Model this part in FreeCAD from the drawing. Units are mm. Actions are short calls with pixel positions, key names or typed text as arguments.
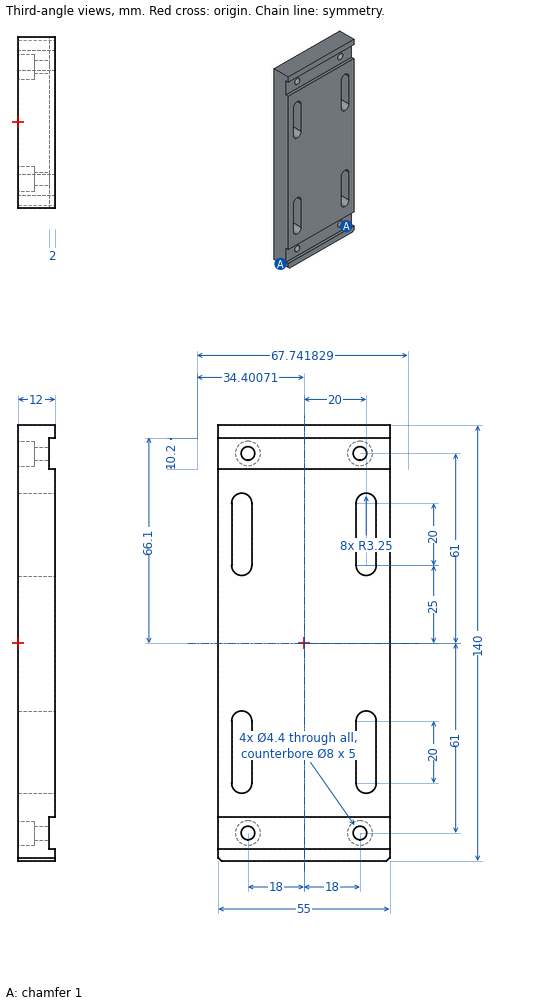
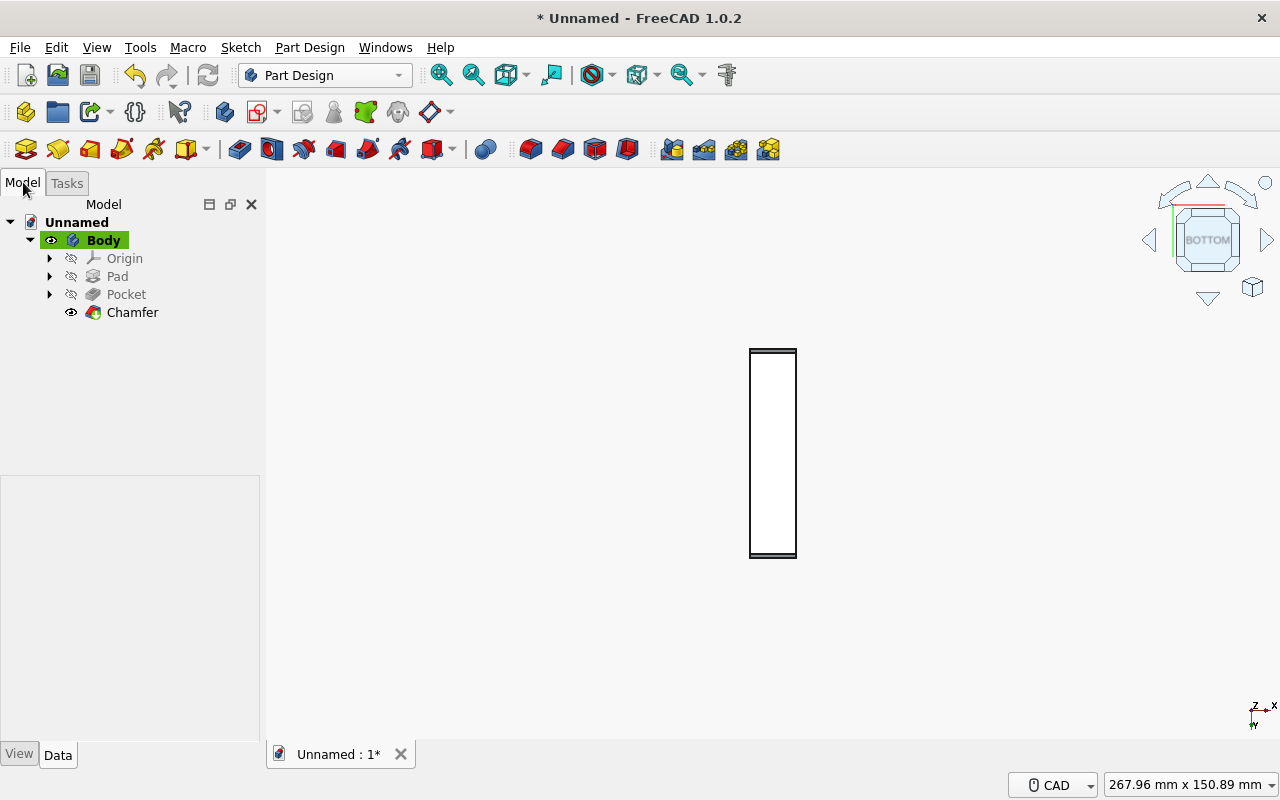
click(116, 294)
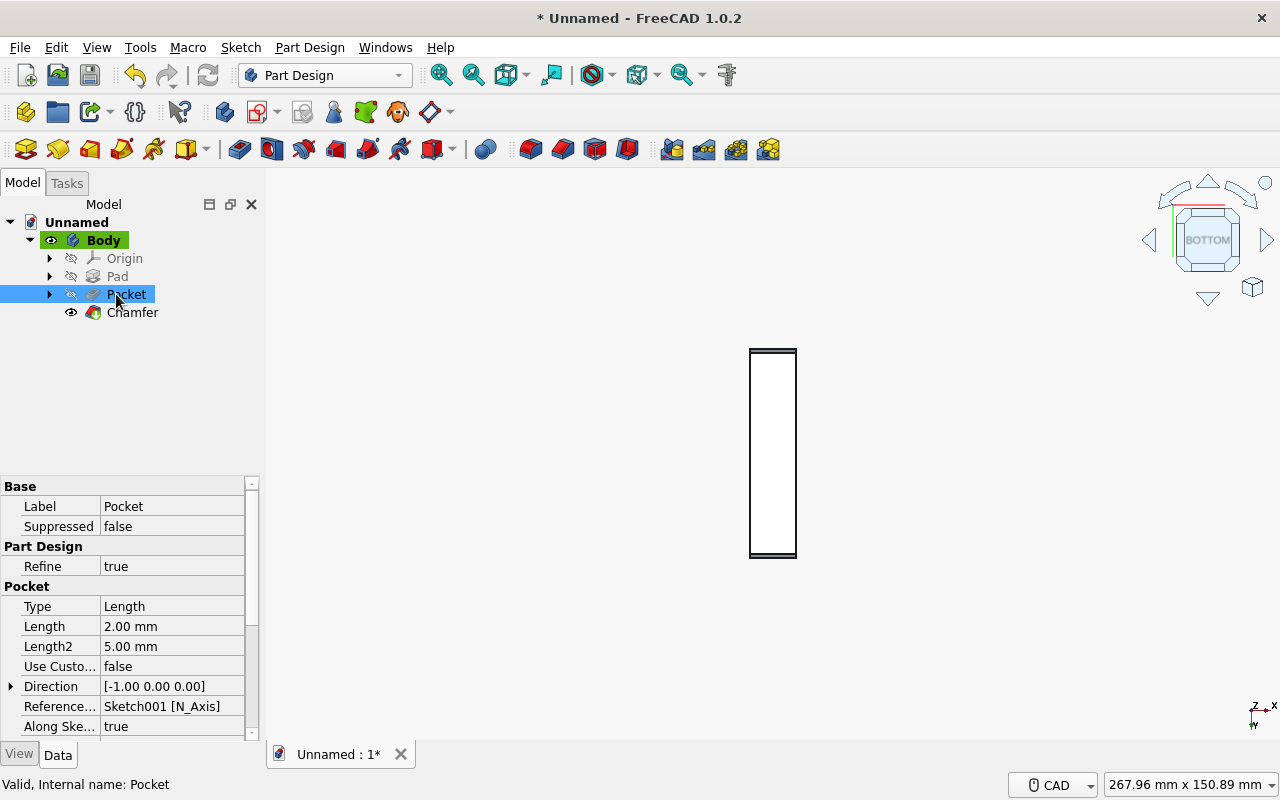
click(672, 150)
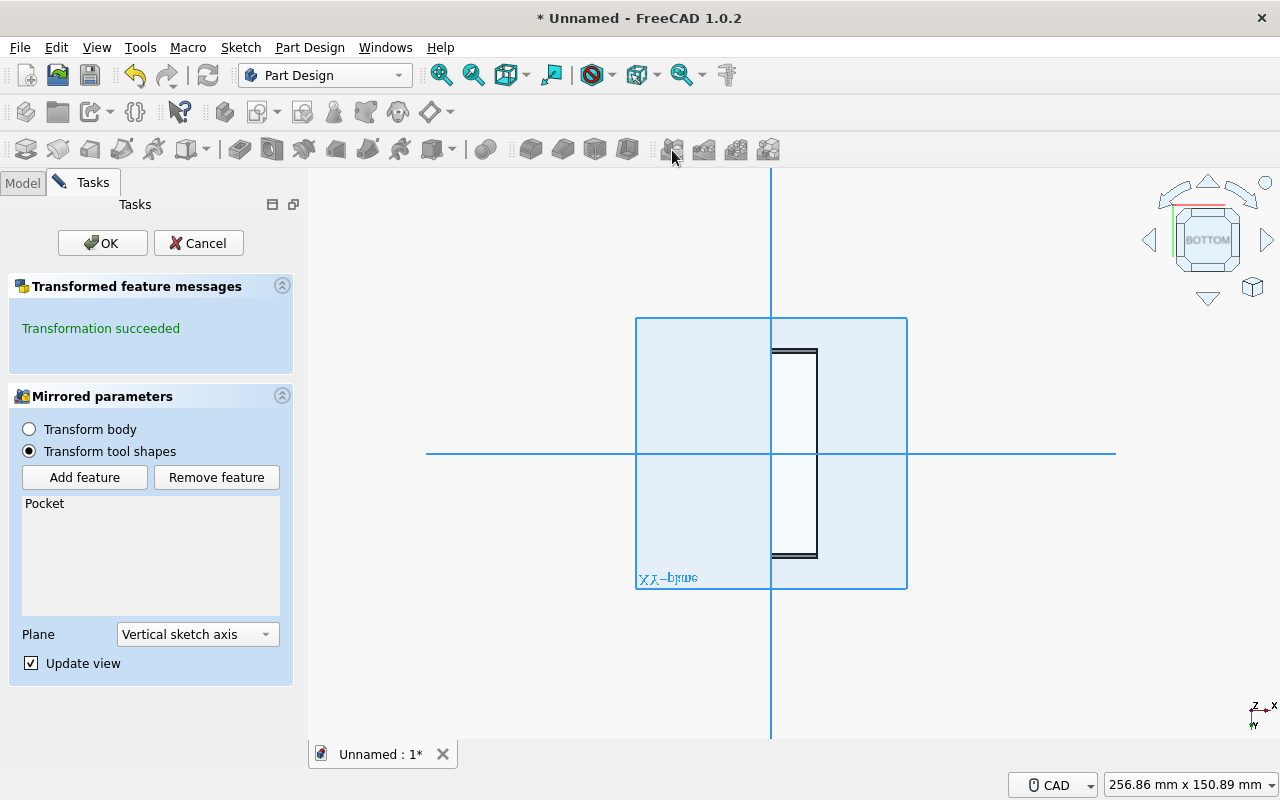
click(198, 634)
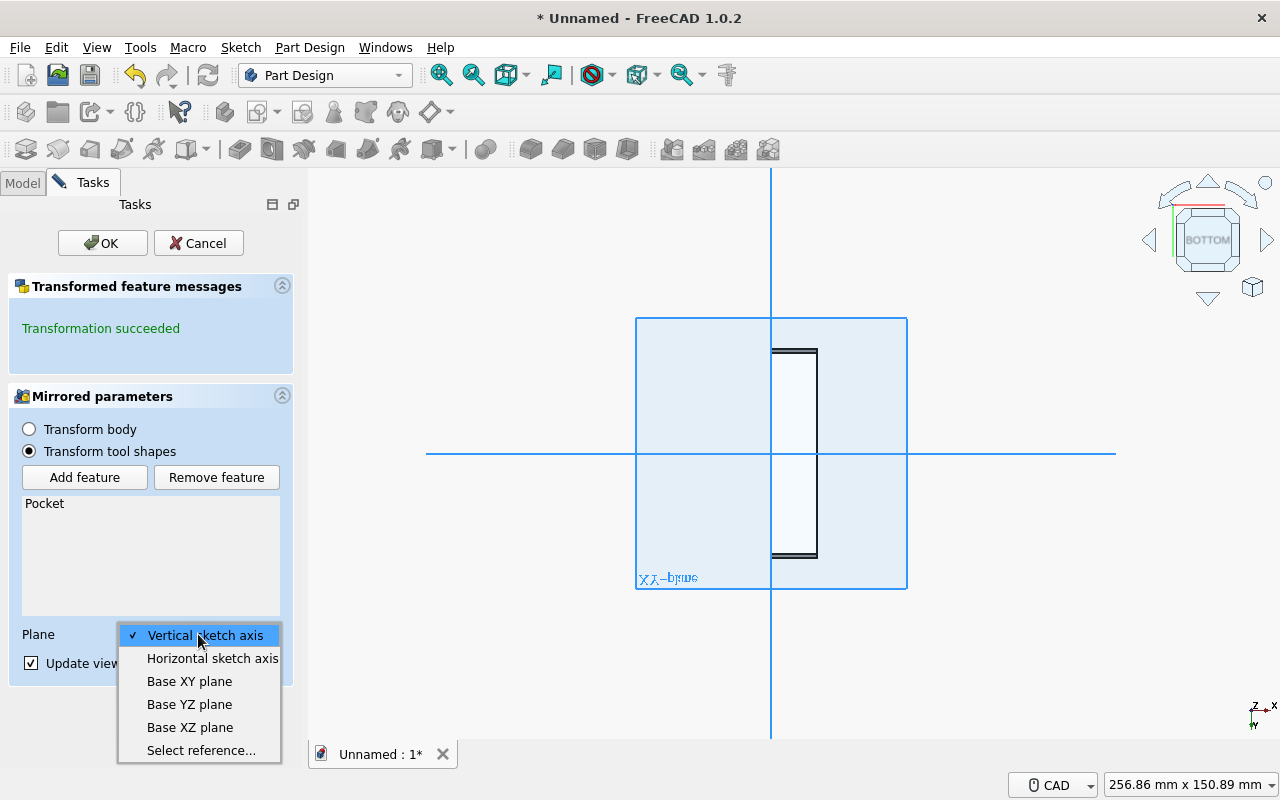
click(198, 682)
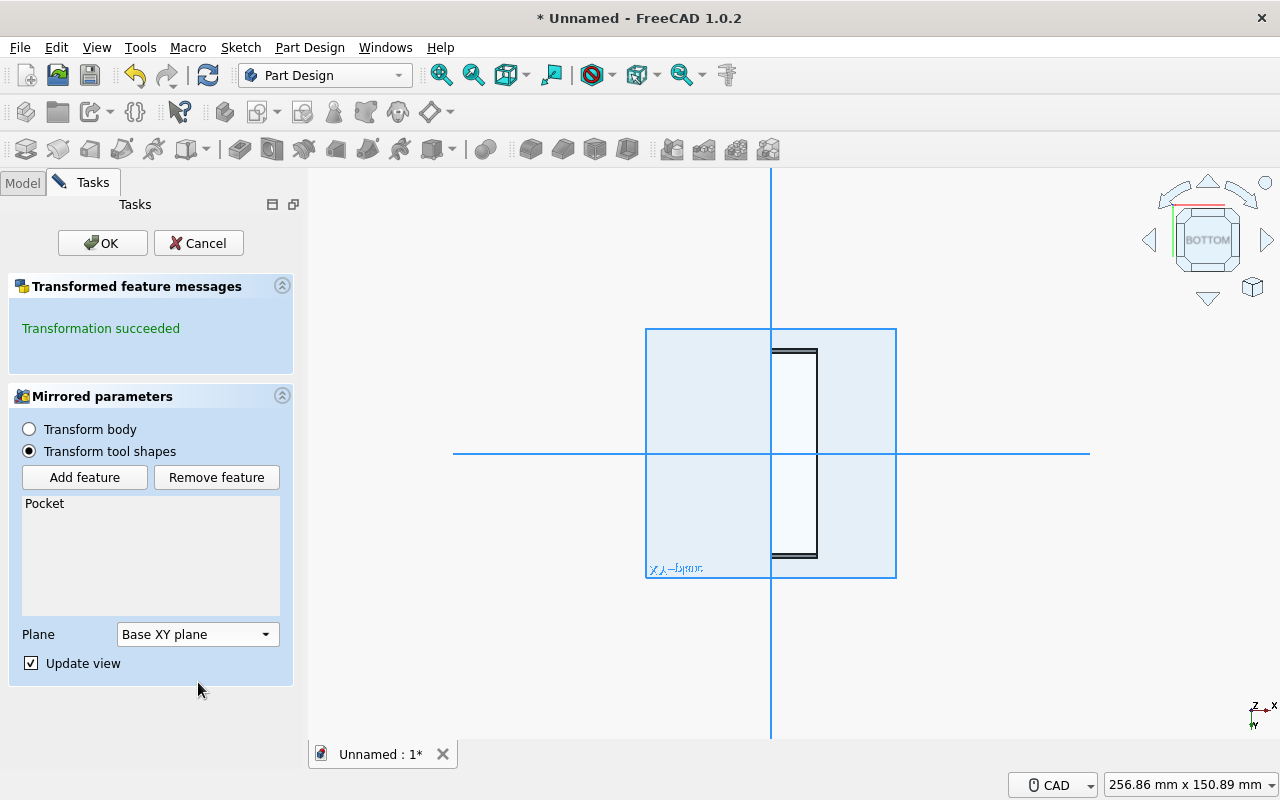
click(103, 243)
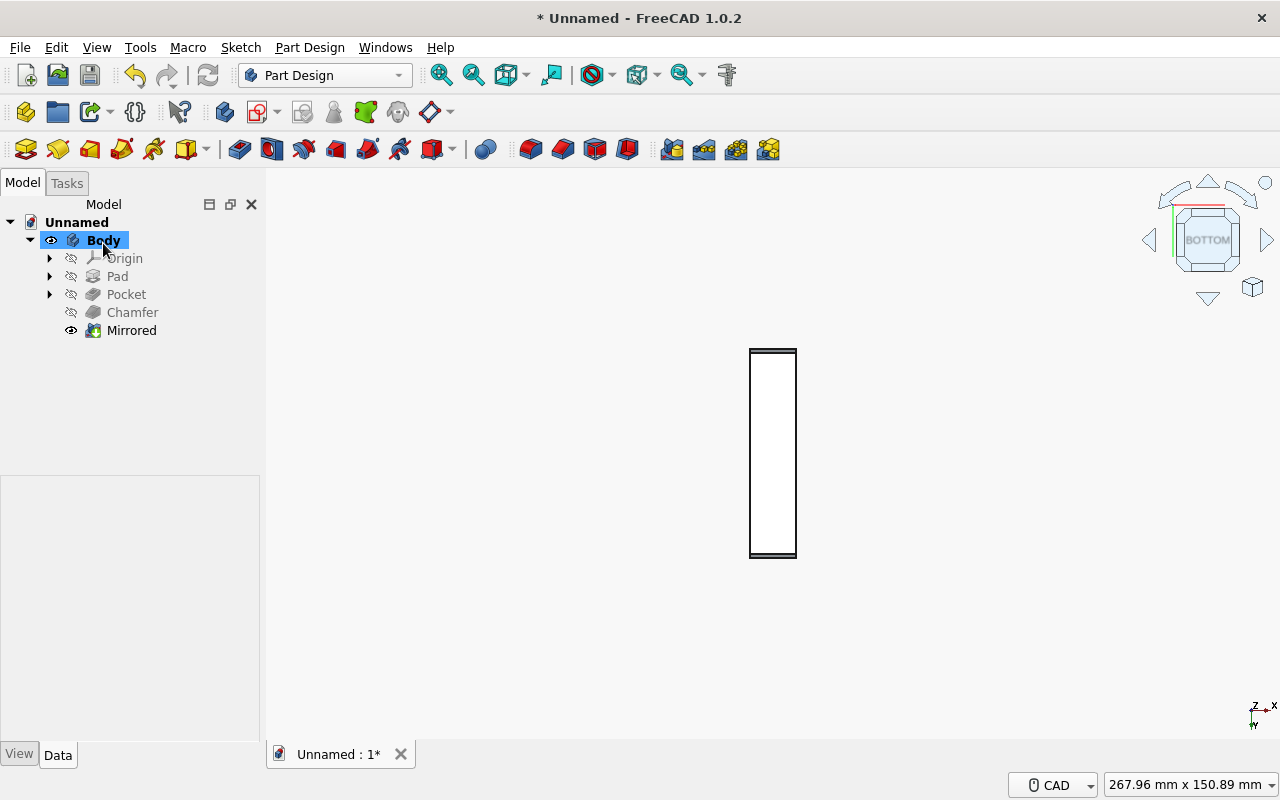
click(442, 76)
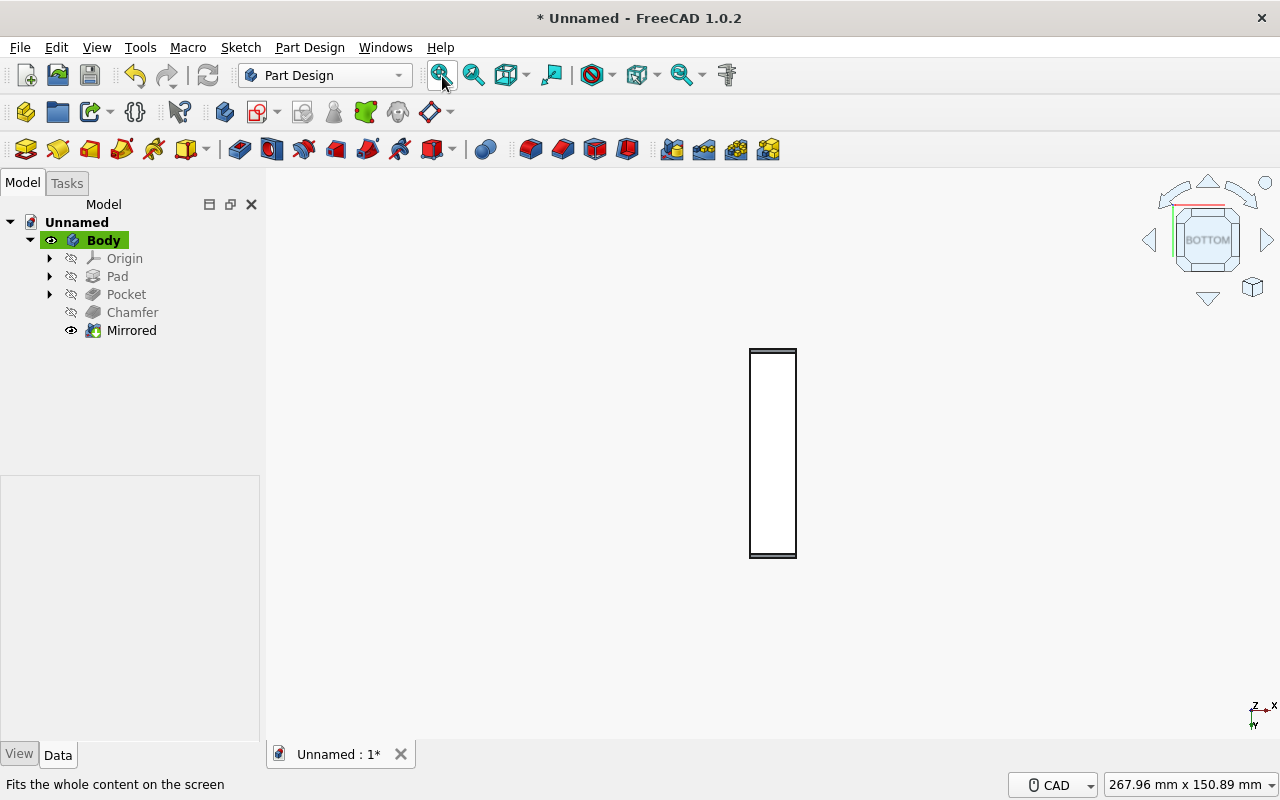
key(0)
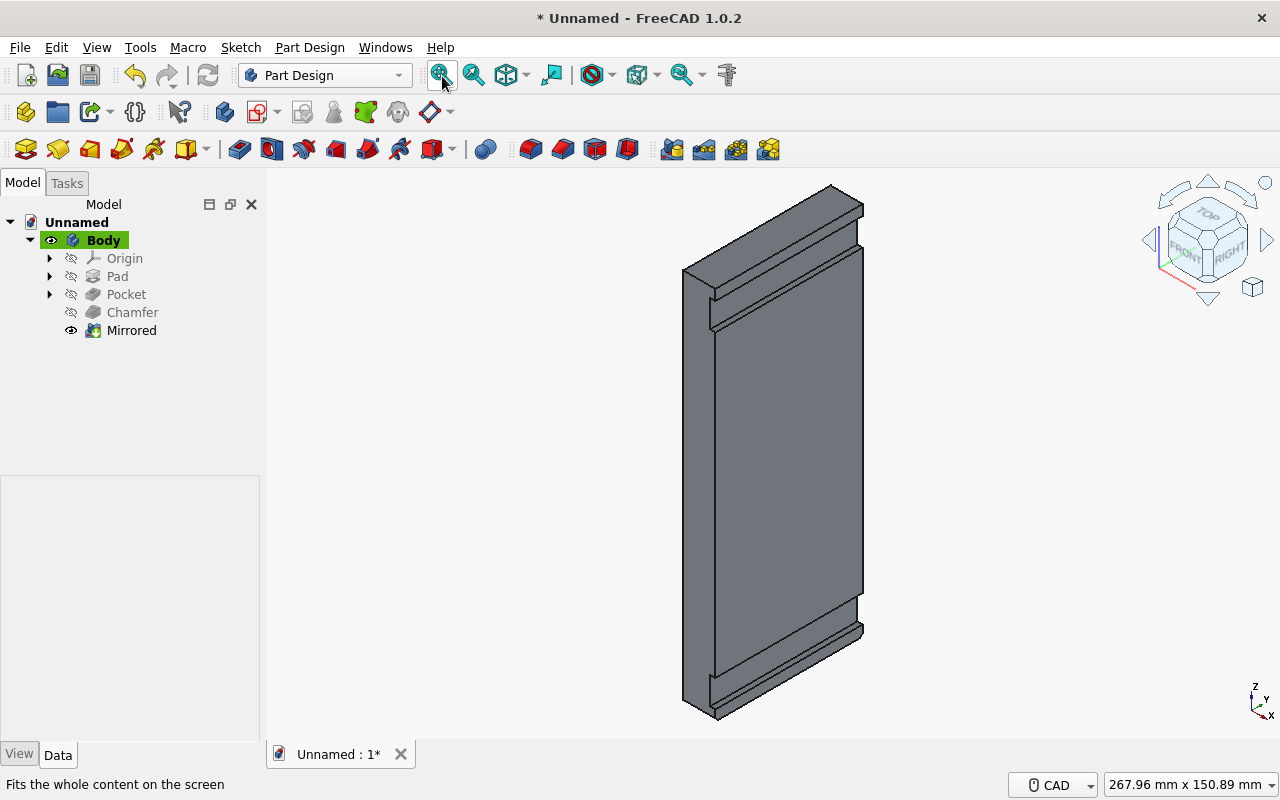
click(789, 511)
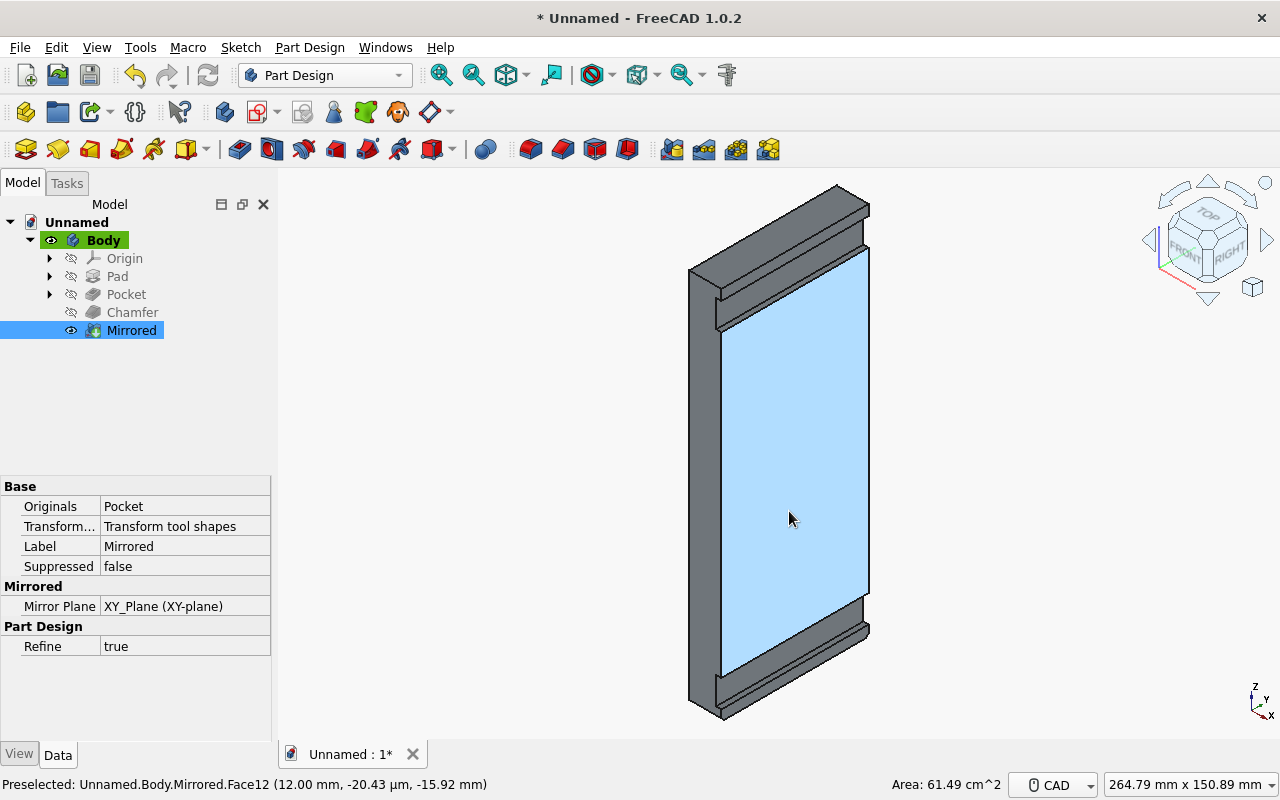
click(258, 112)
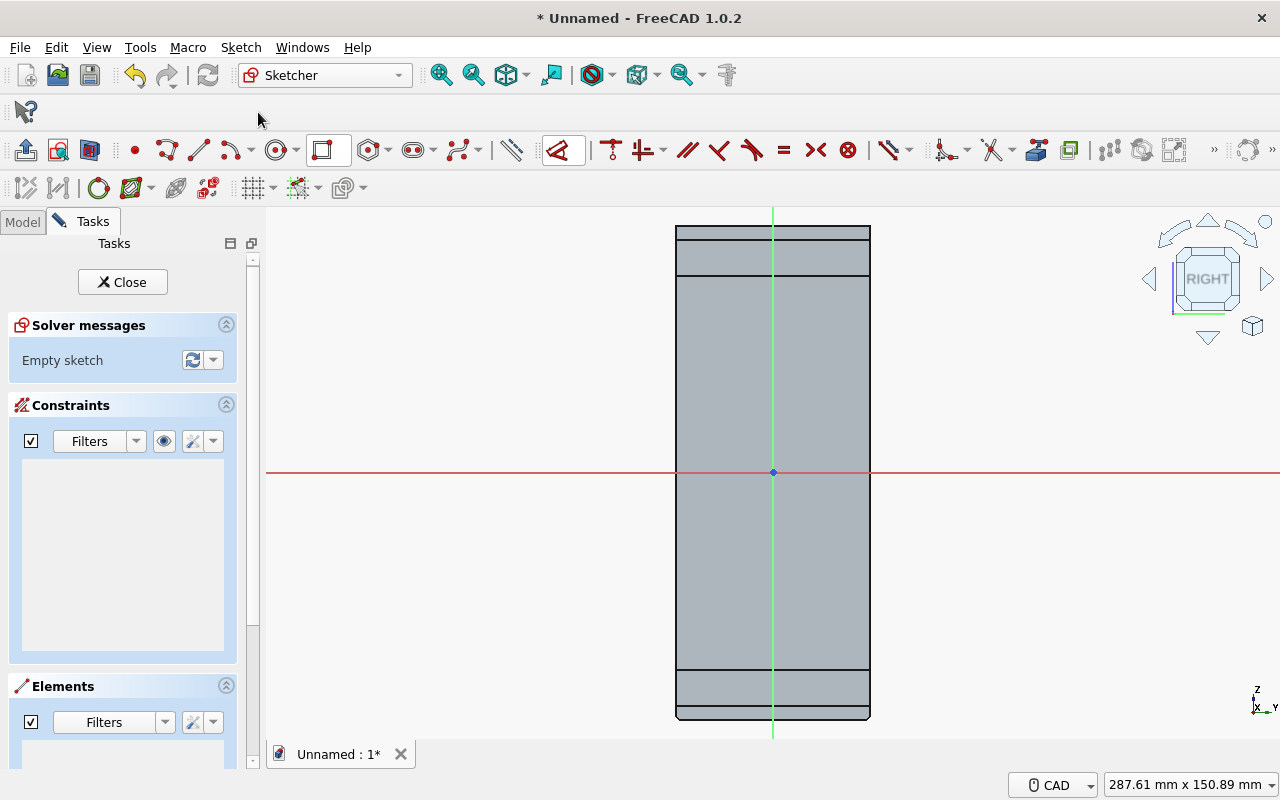
click(414, 150)